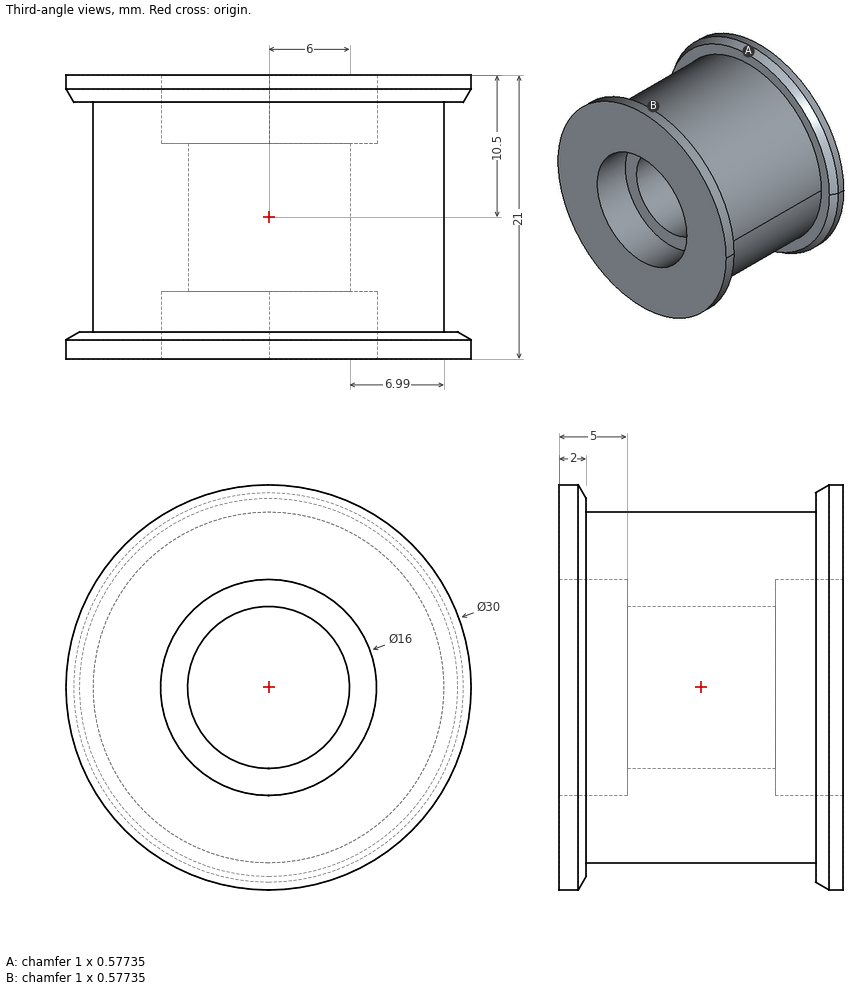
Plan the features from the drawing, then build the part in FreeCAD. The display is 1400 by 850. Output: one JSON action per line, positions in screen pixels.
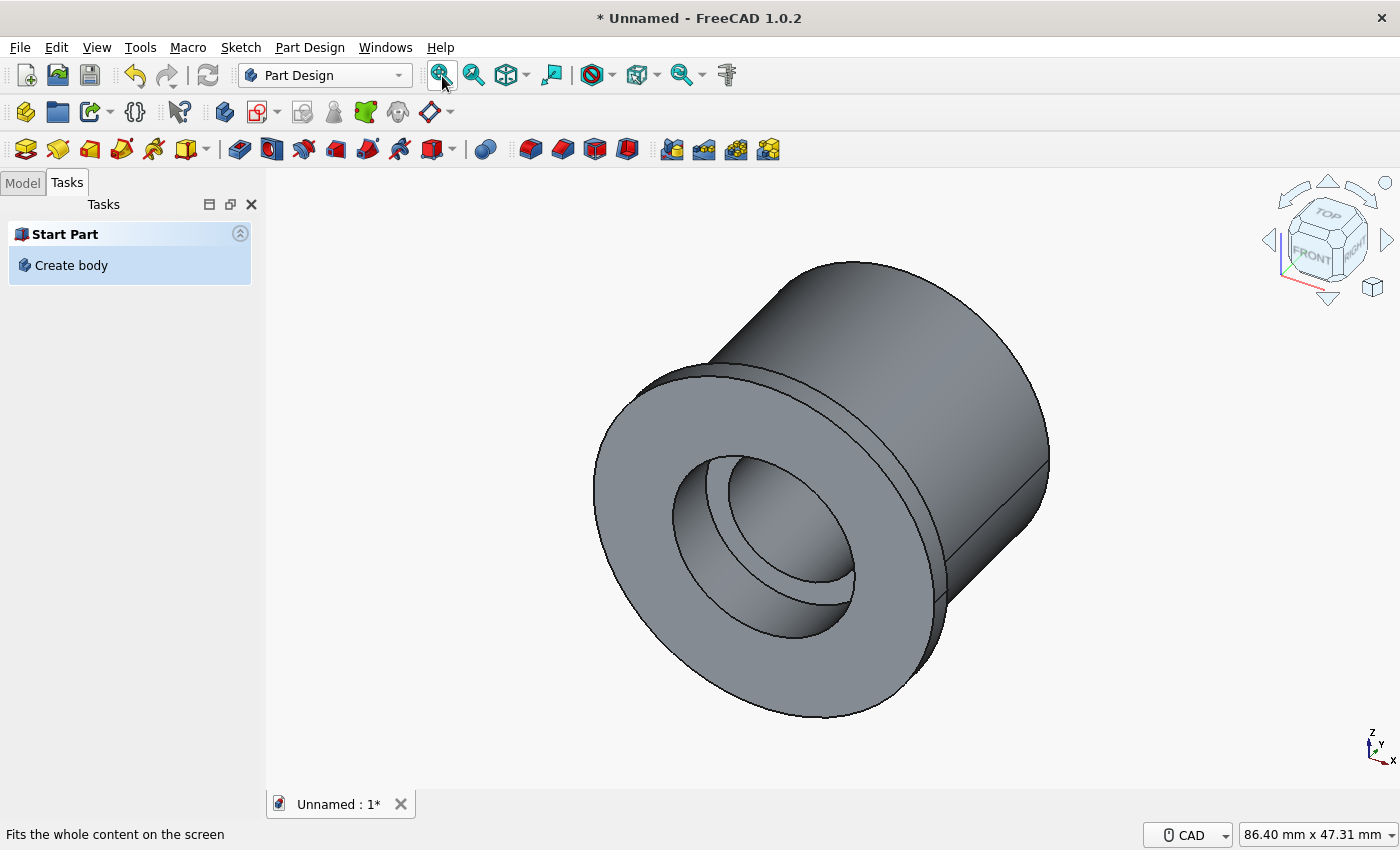
{"action": "left_click", "coordinate": [23, 182]}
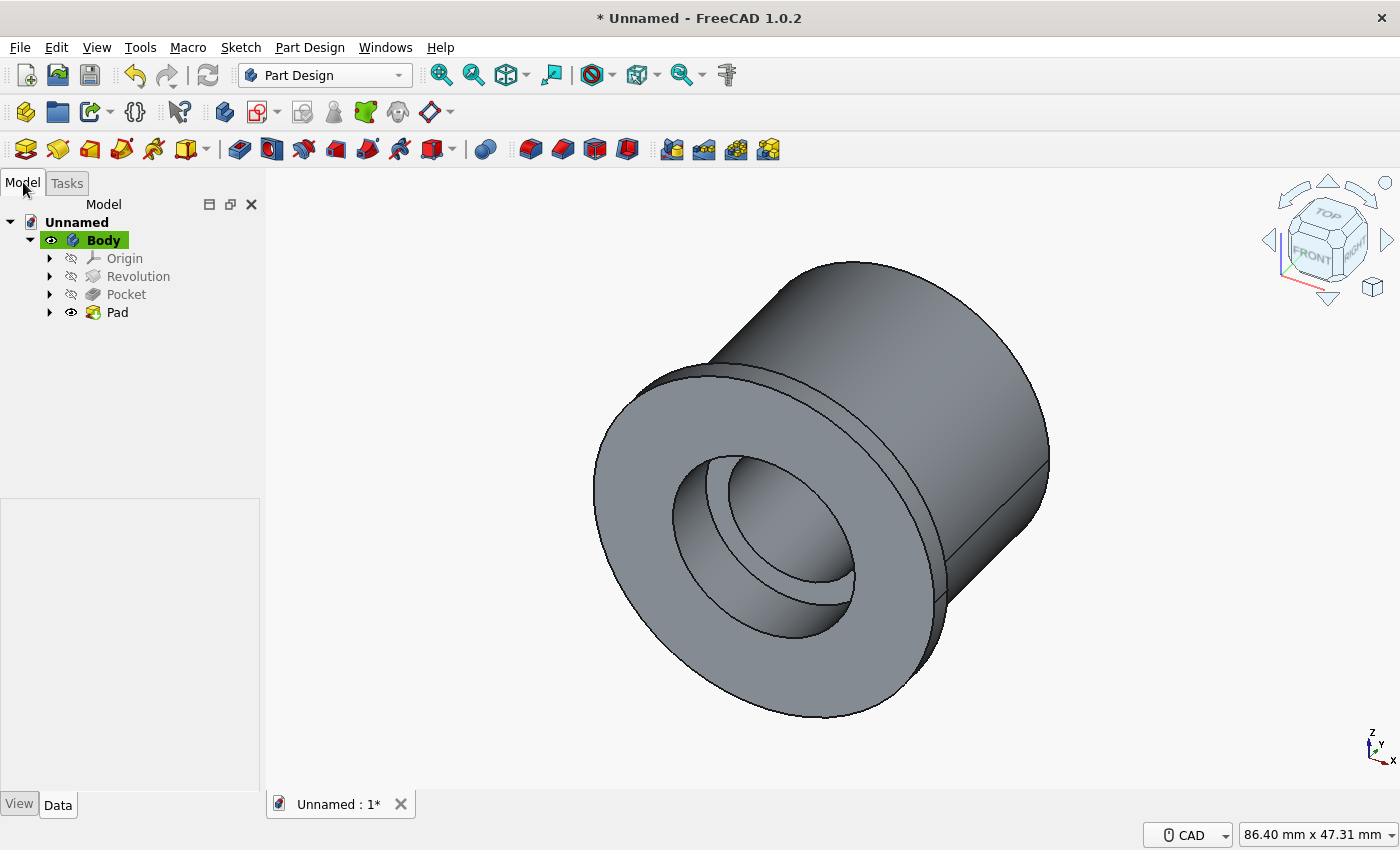
{"action": "left_click", "coordinate": [116, 294]}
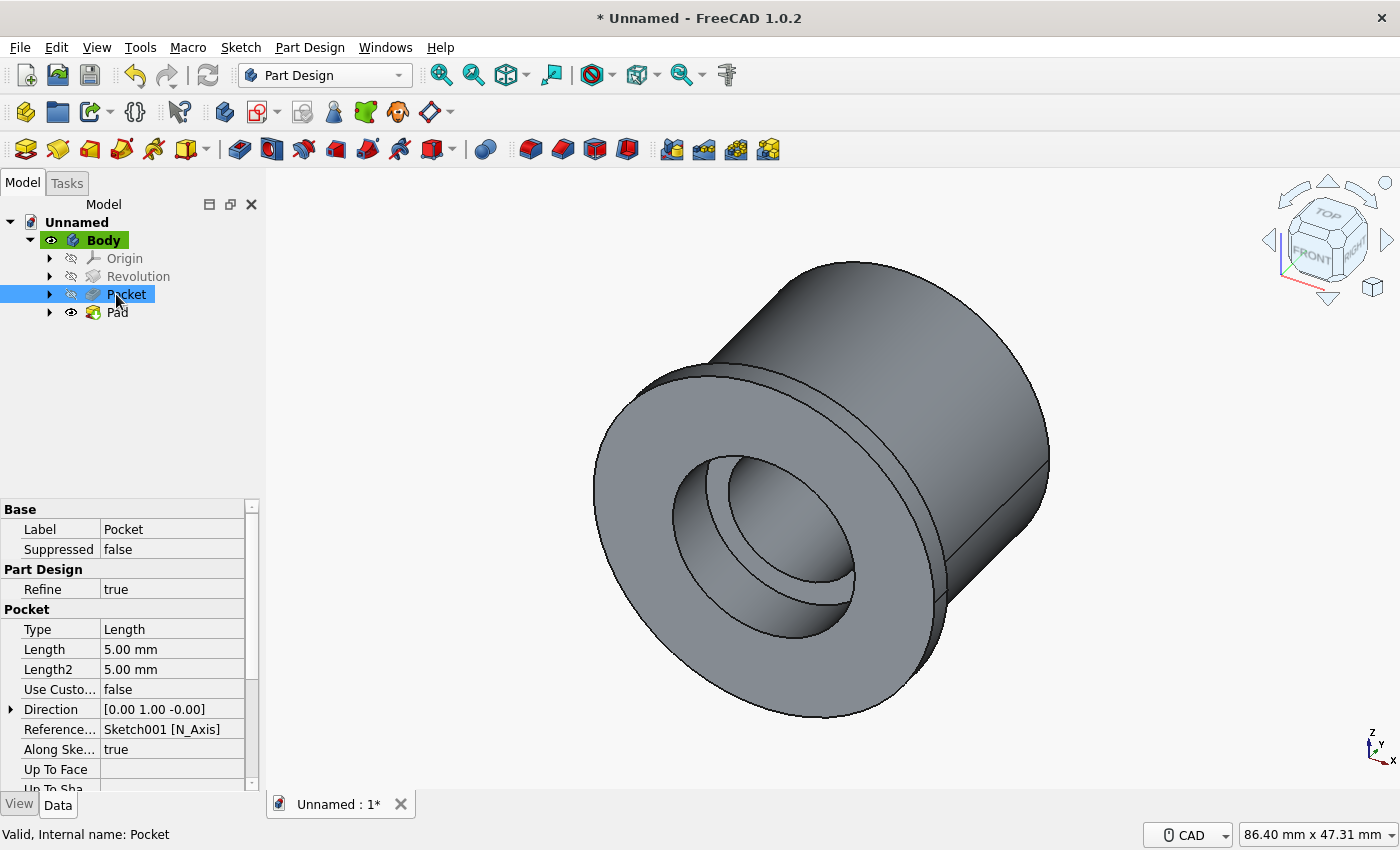
{"action": "left_click", "coordinate": [116, 312], "text": "ctrl"}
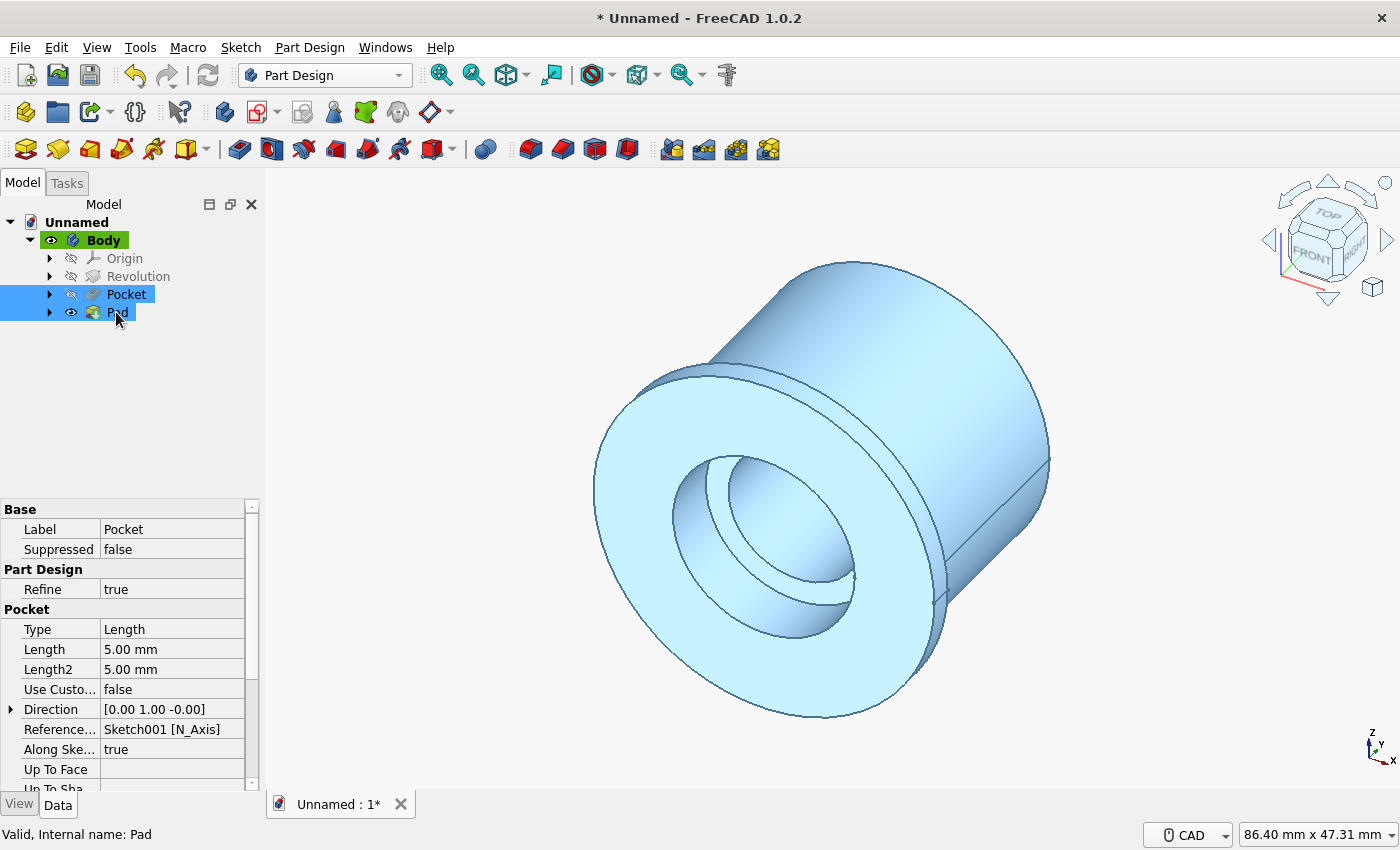
{"action": "left_click", "coordinate": [672, 150]}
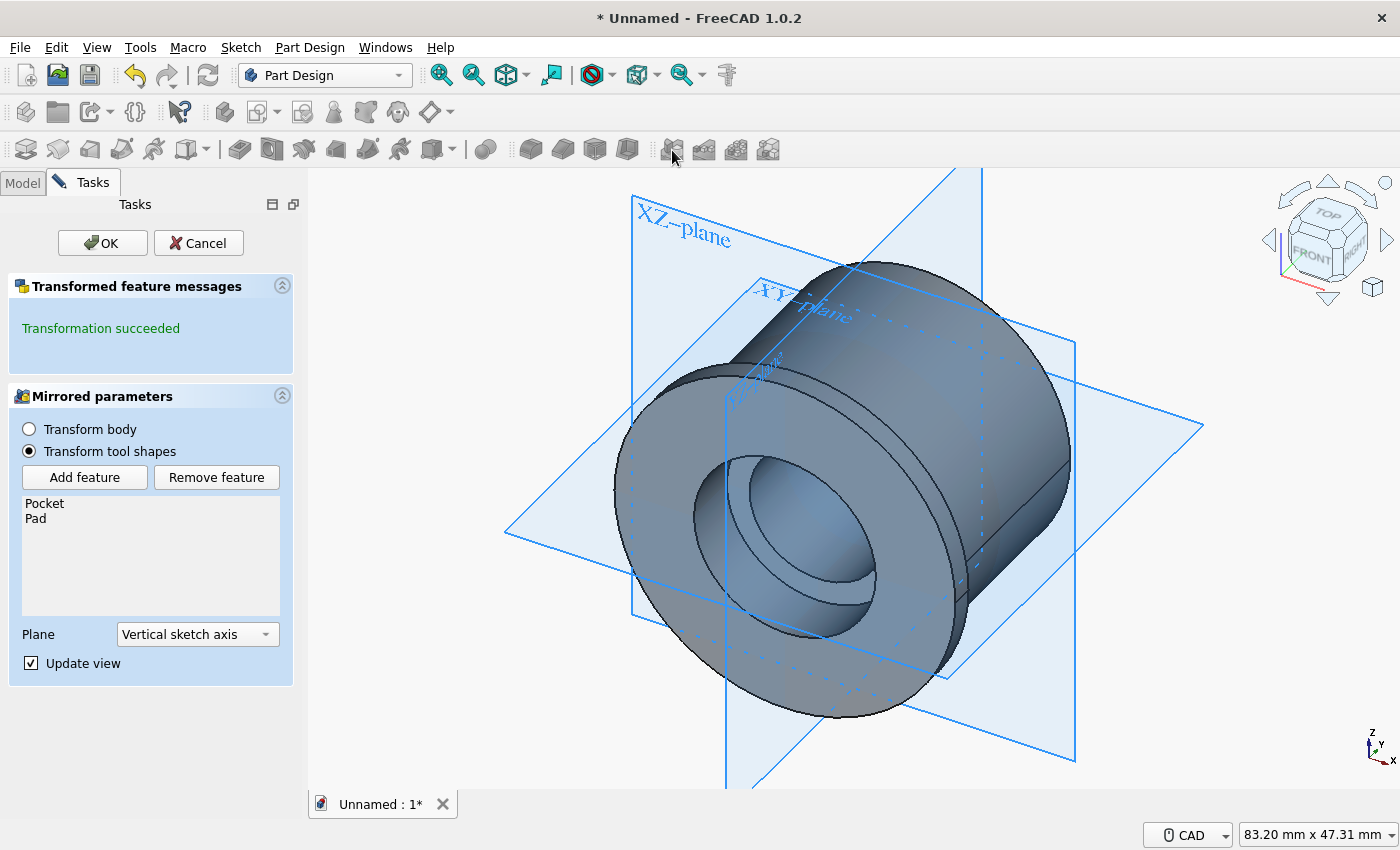
{"action": "left_click", "coordinate": [198, 634]}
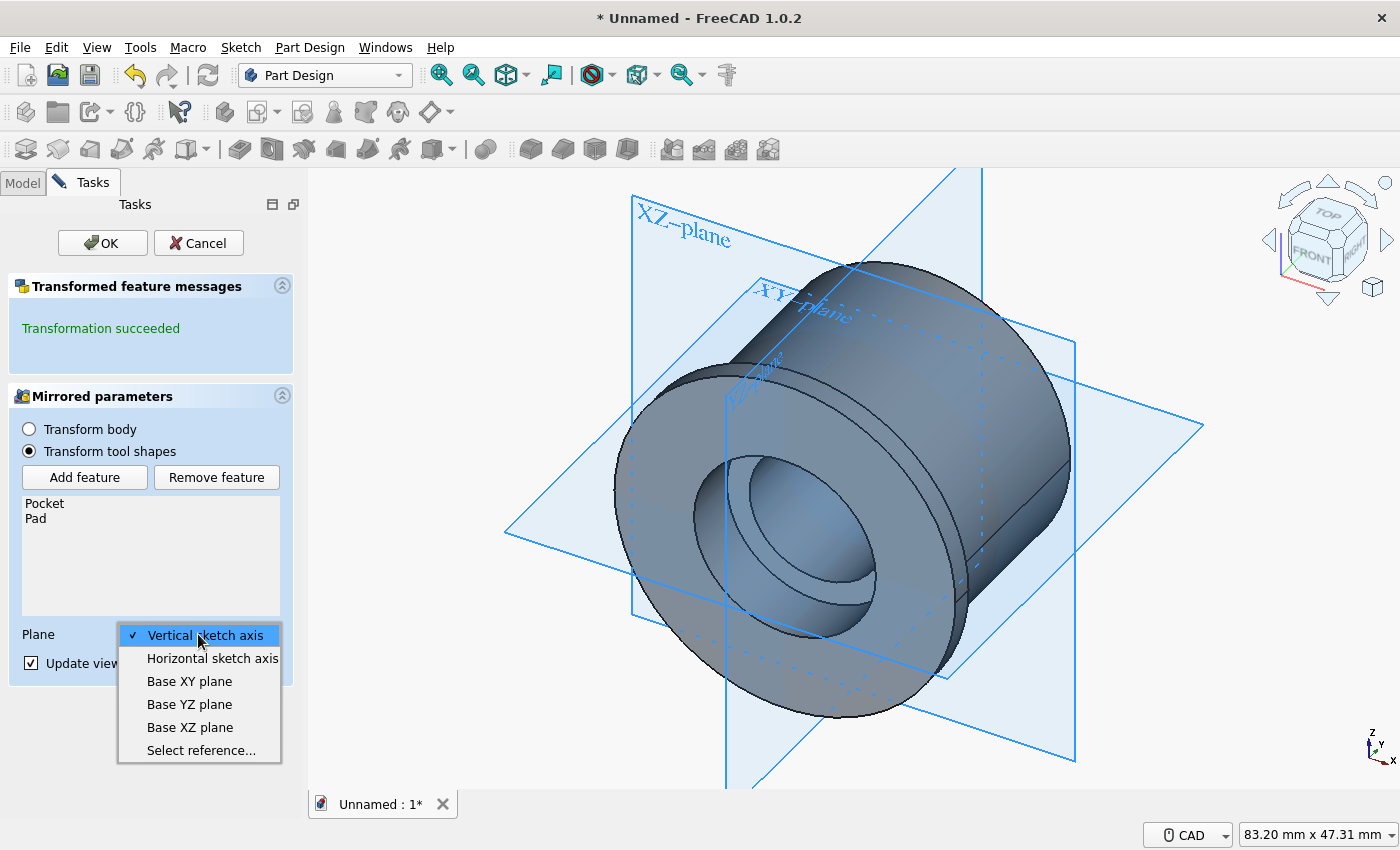
{"action": "left_click", "coordinate": [198, 728]}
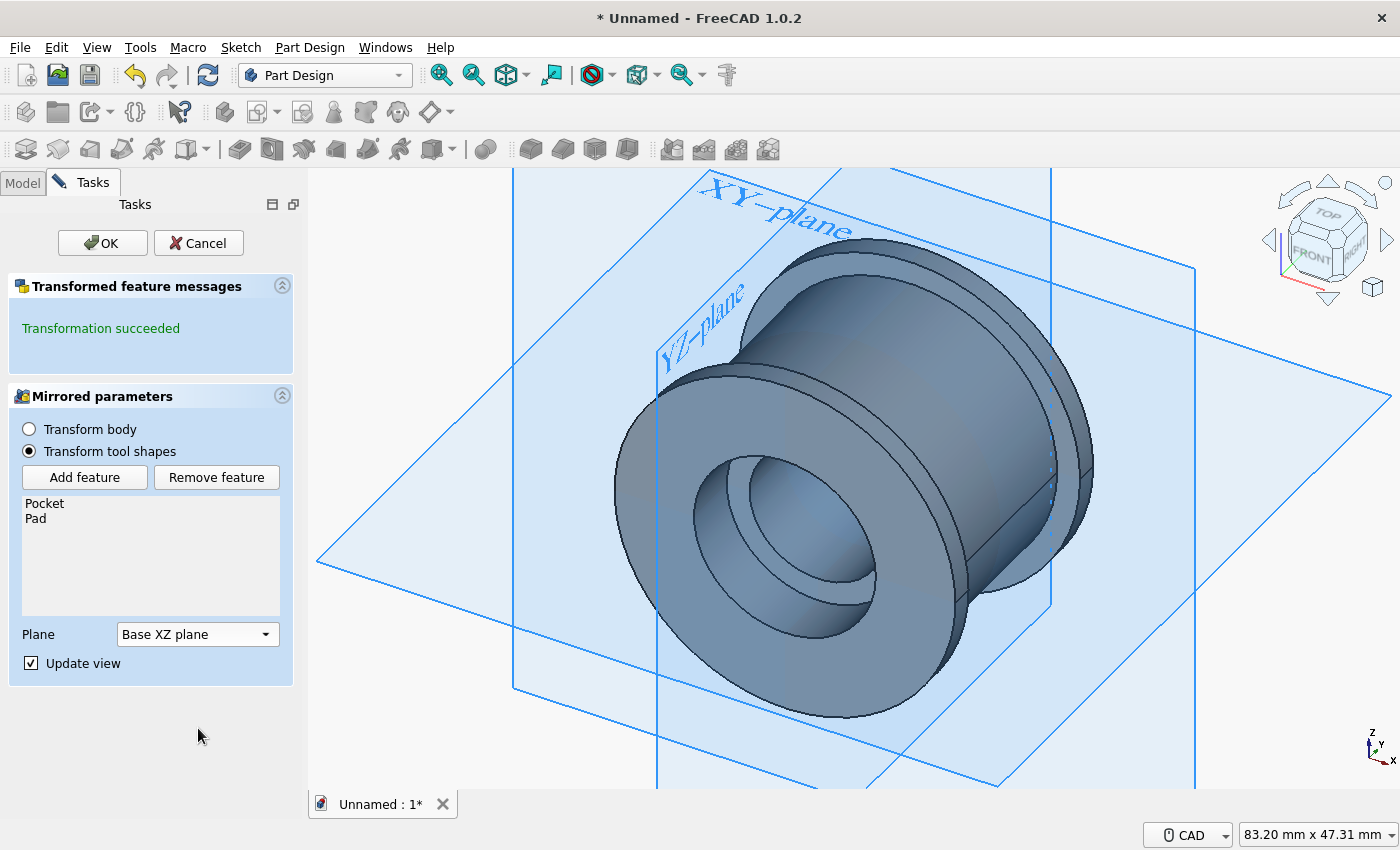
{"action": "left_click", "coordinate": [103, 243]}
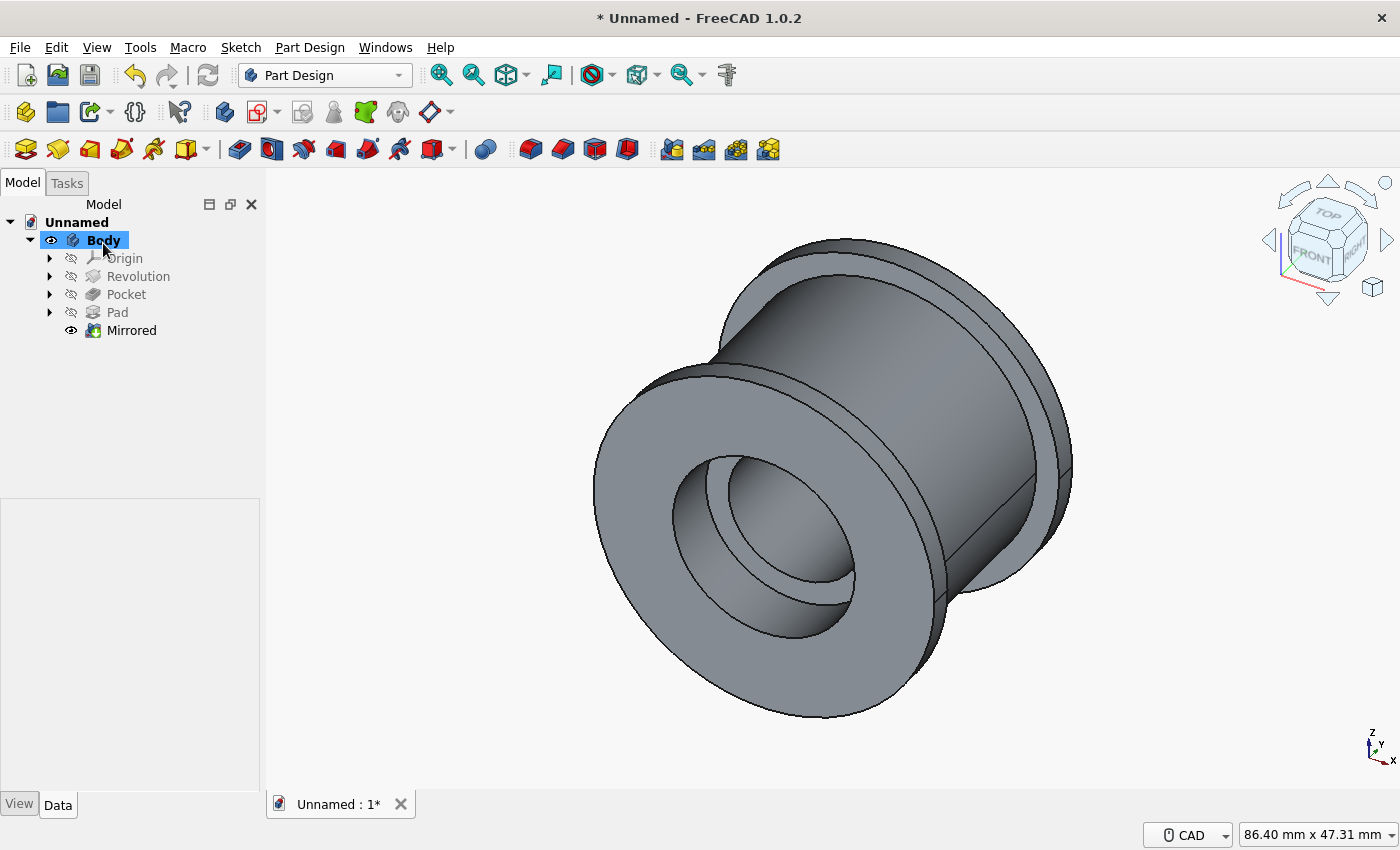
{"action": "left_click", "coordinate": [836, 251]}